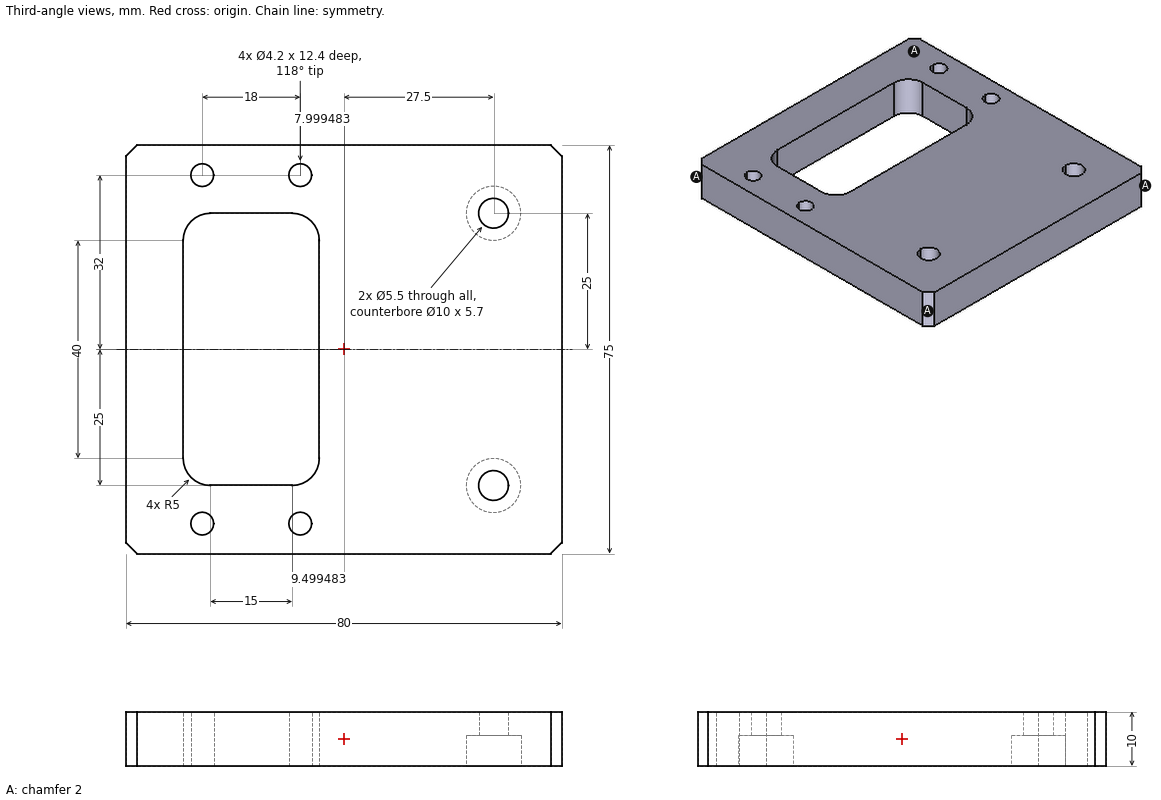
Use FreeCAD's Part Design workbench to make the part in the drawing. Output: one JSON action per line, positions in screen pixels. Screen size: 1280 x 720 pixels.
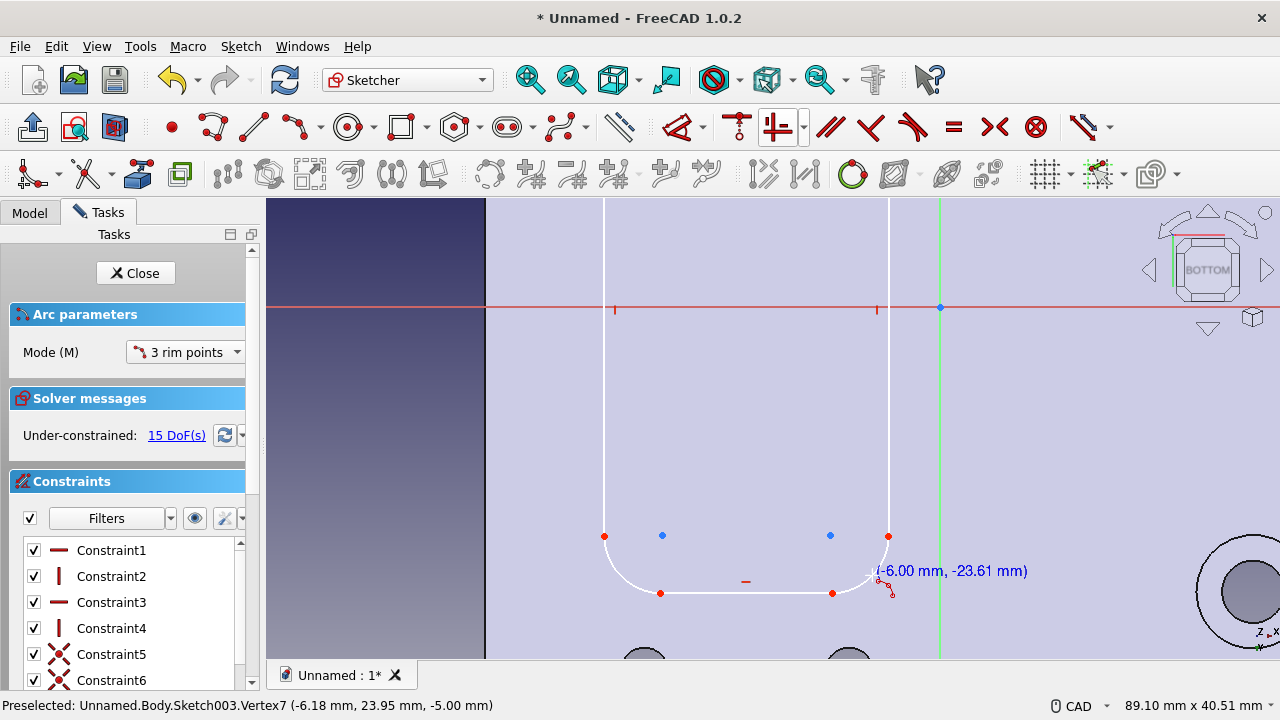
{"action": "scroll", "coordinate": [622, 576], "scroll_direction": "down", "scroll_amount": 3}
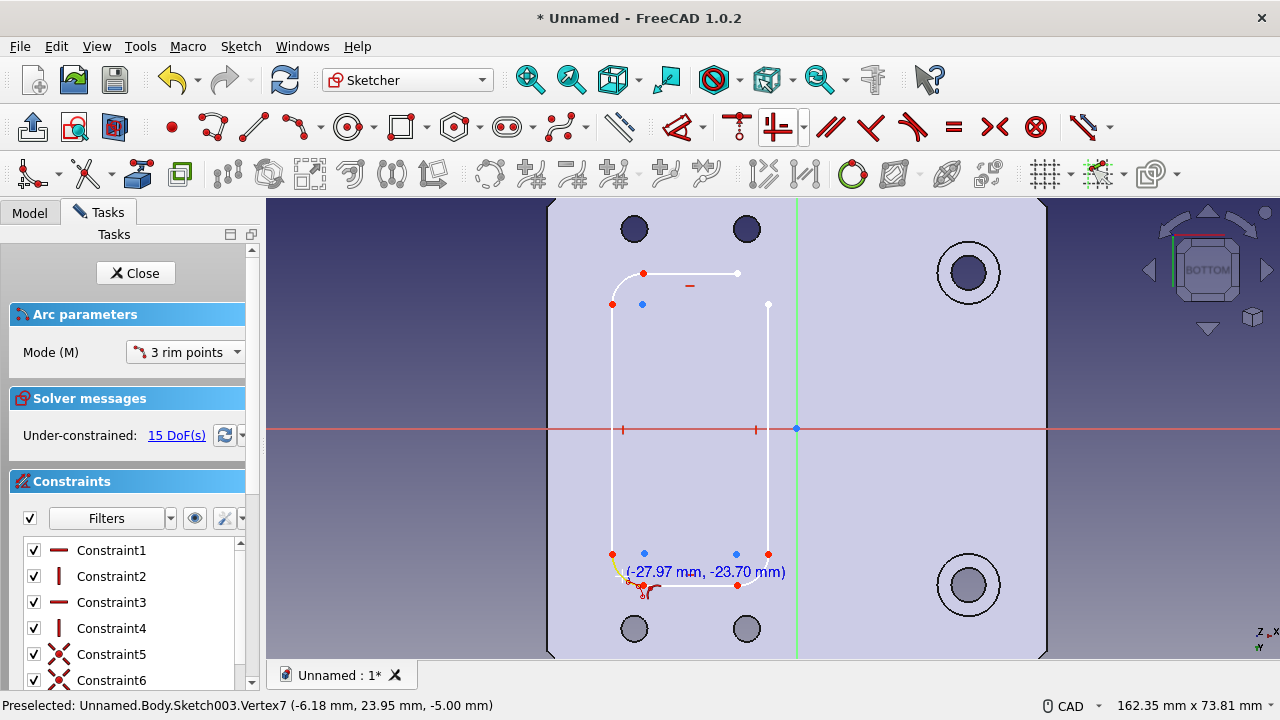
{"action": "left_click", "coordinate": [768, 305]}
{"action": "left_click", "coordinate": [737, 274]}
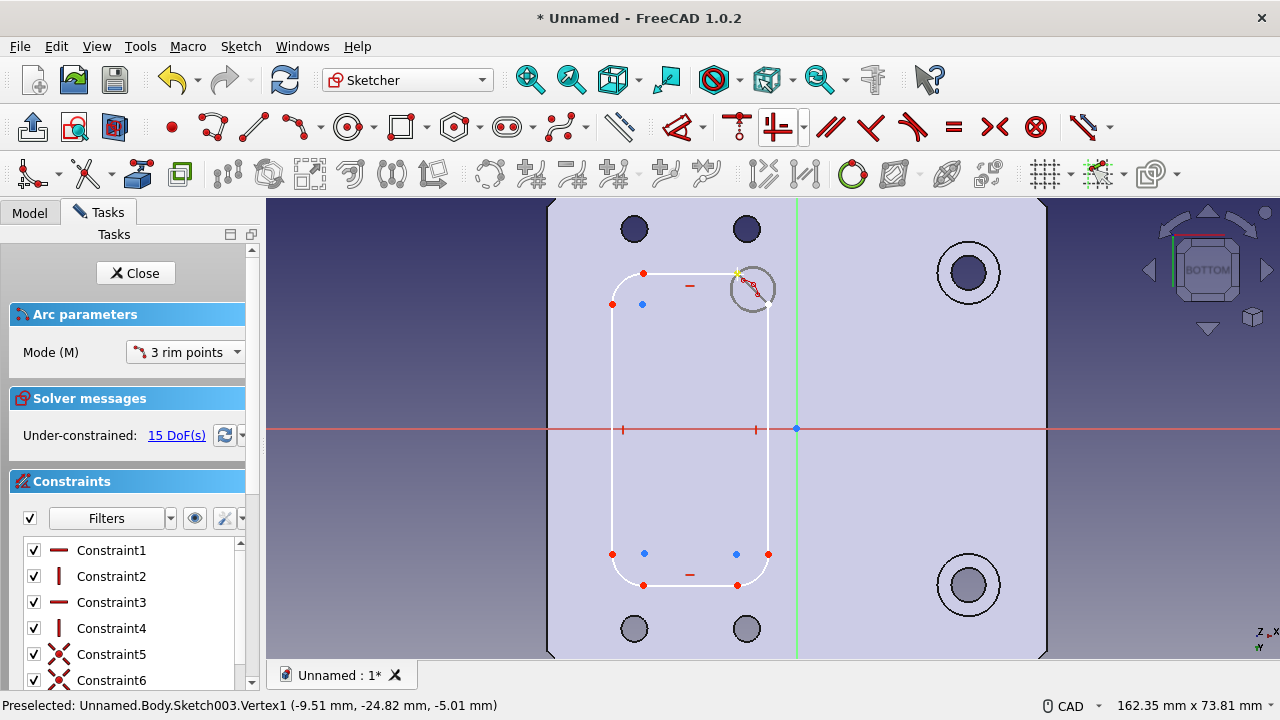
{"action": "scroll", "coordinate": [760, 282], "scroll_direction": "up", "scroll_amount": 3}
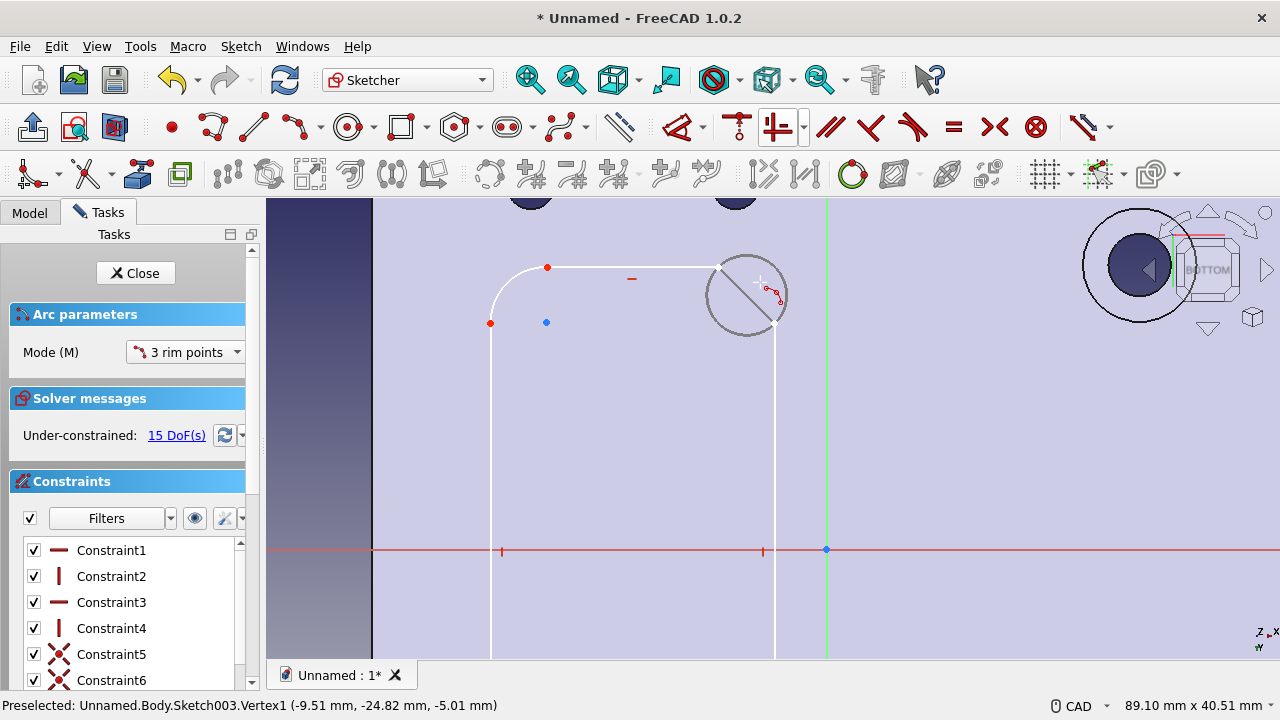
{"action": "left_click", "coordinate": [759, 282]}
{"action": "key", "text": "Escape"}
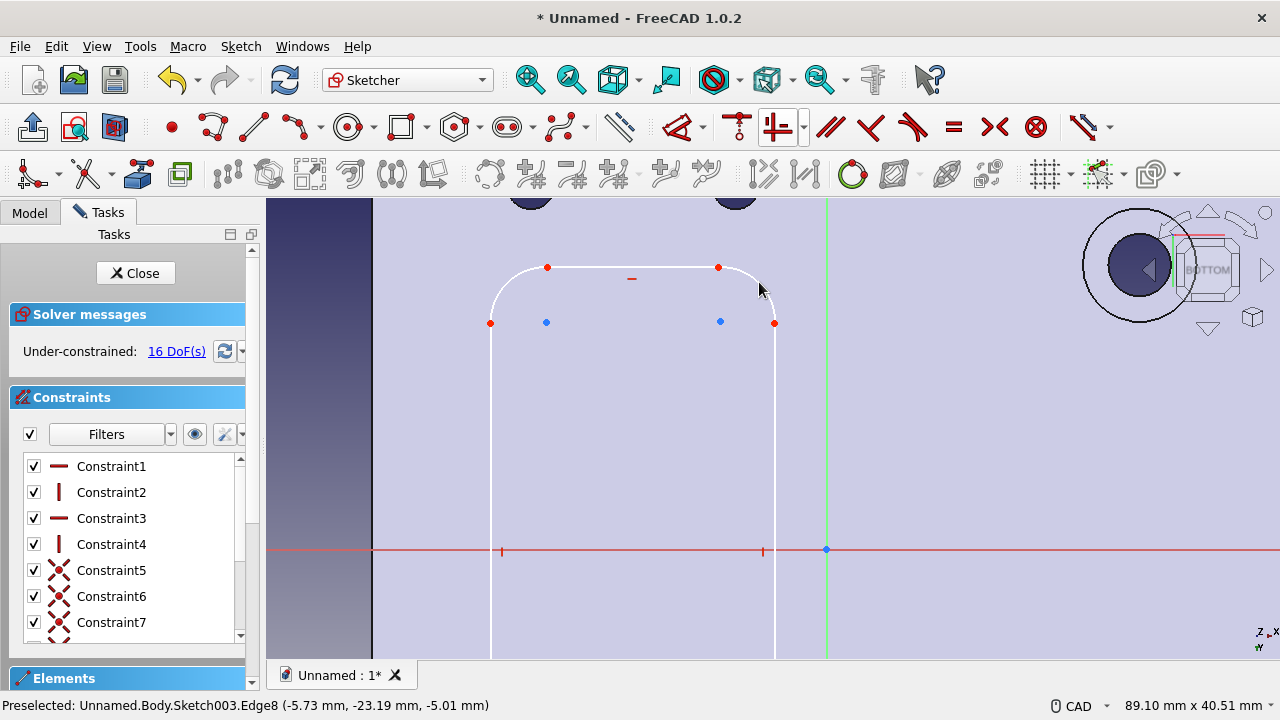
{"action": "left_click", "coordinate": [667, 267]}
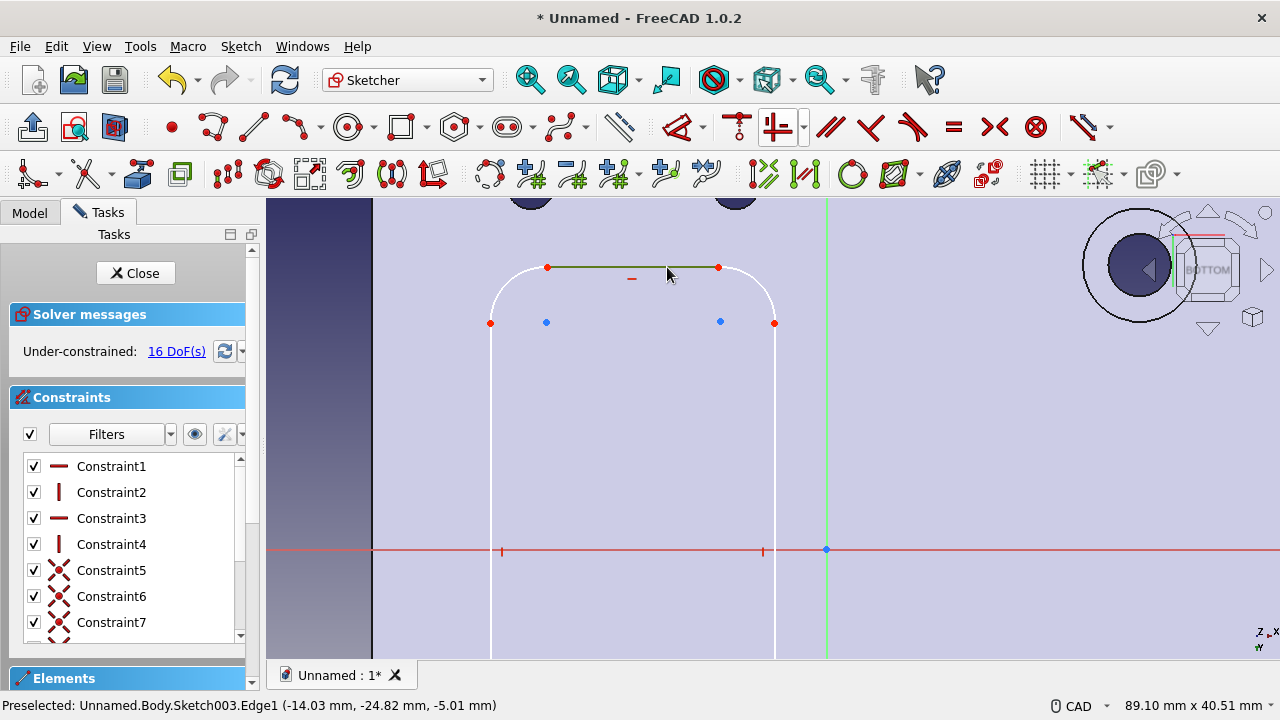
{"action": "left_click", "coordinate": [521, 273]}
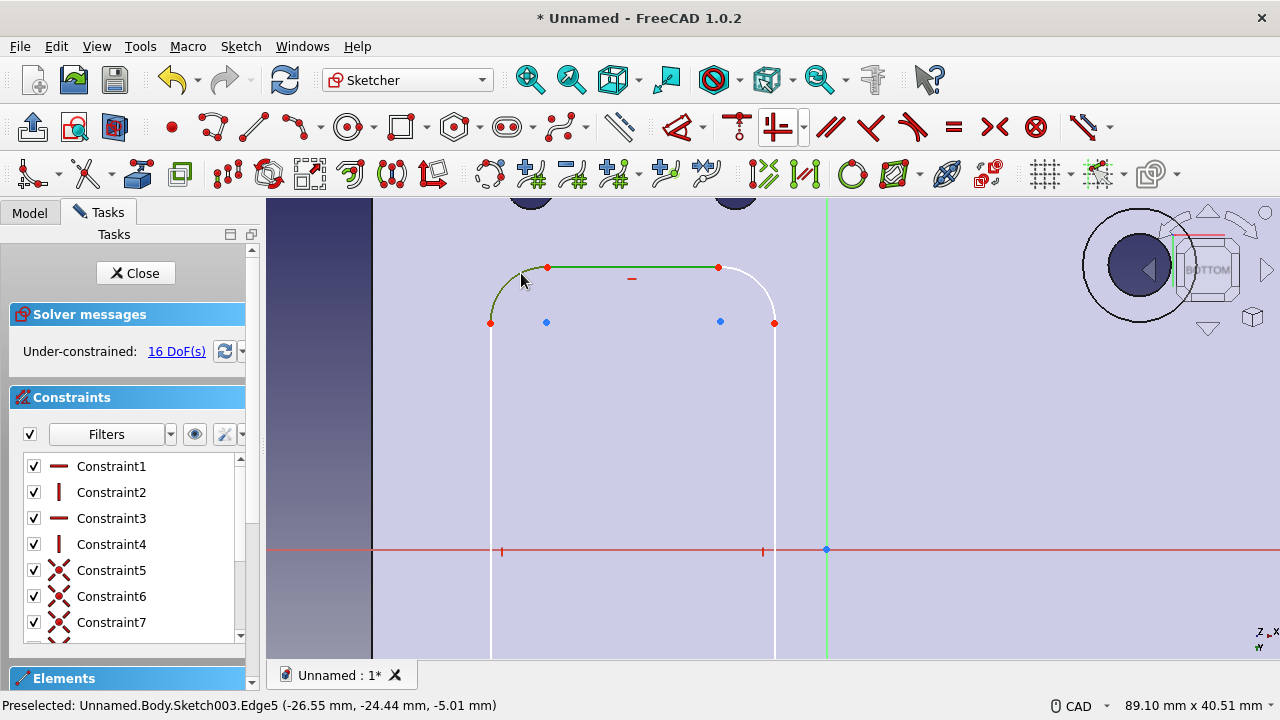
{"action": "key", "text": "t"}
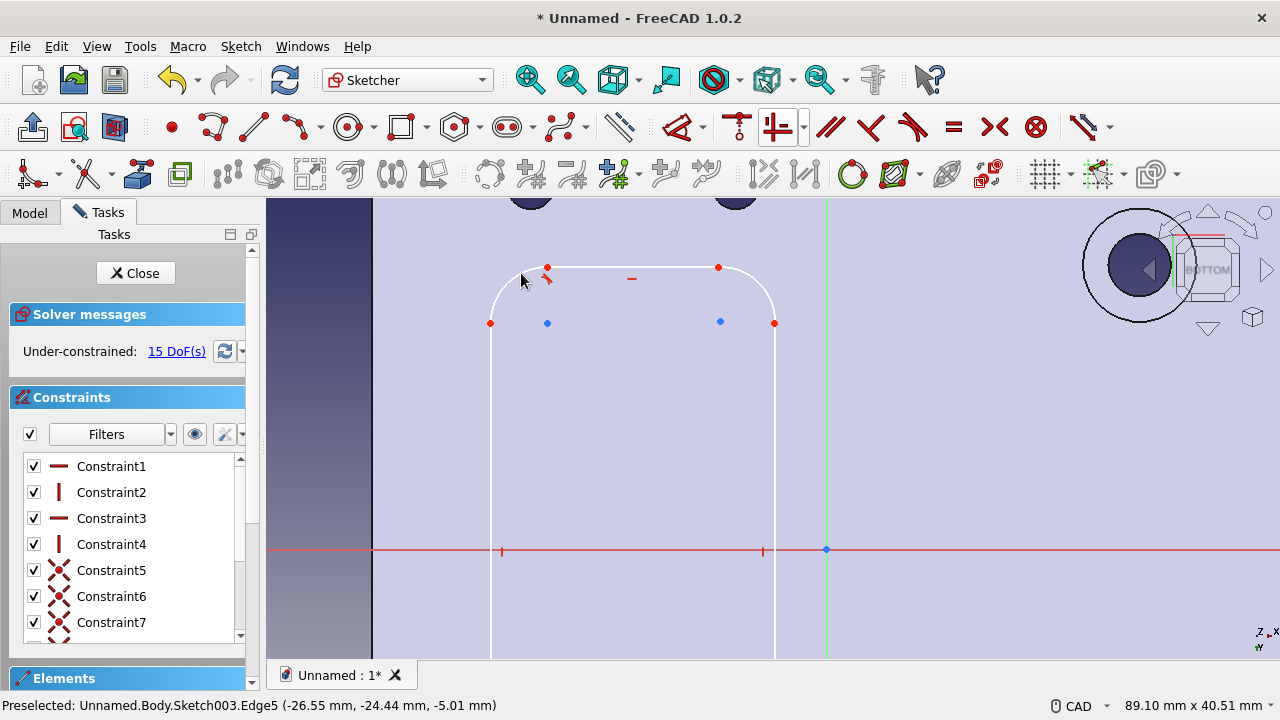
{"action": "left_click", "coordinate": [667, 267]}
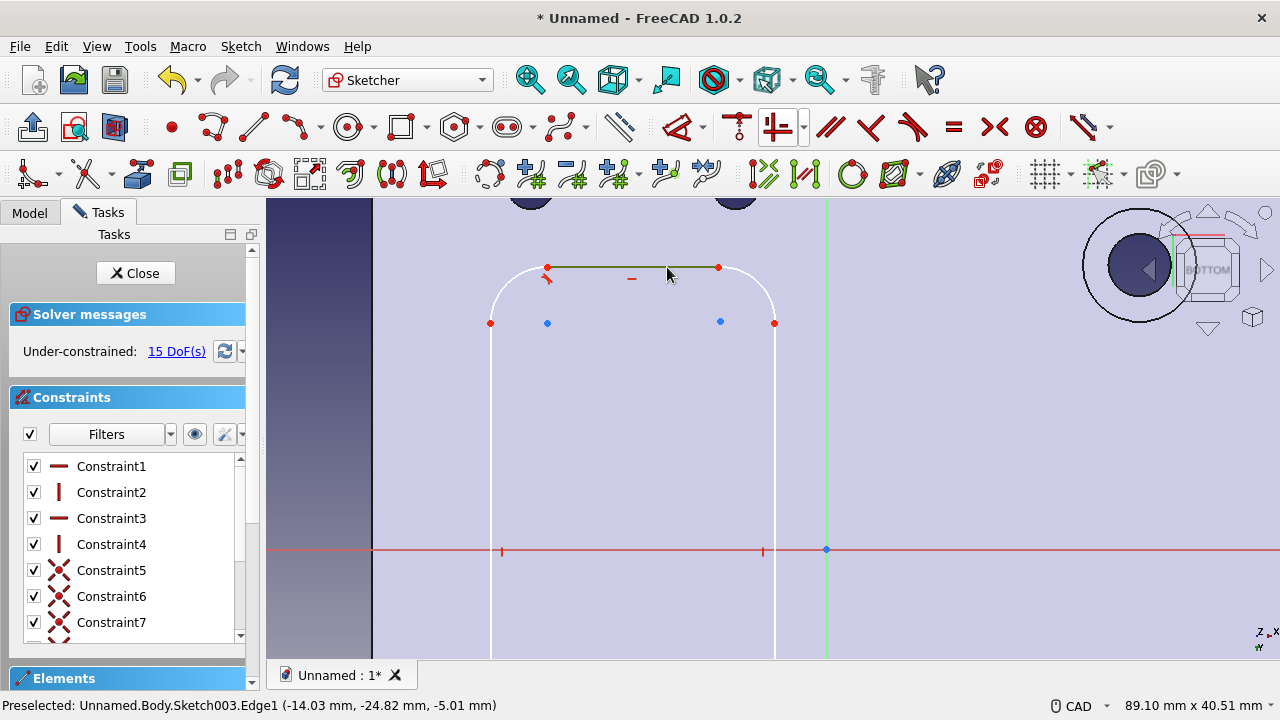
{"action": "left_click", "coordinate": [769, 298]}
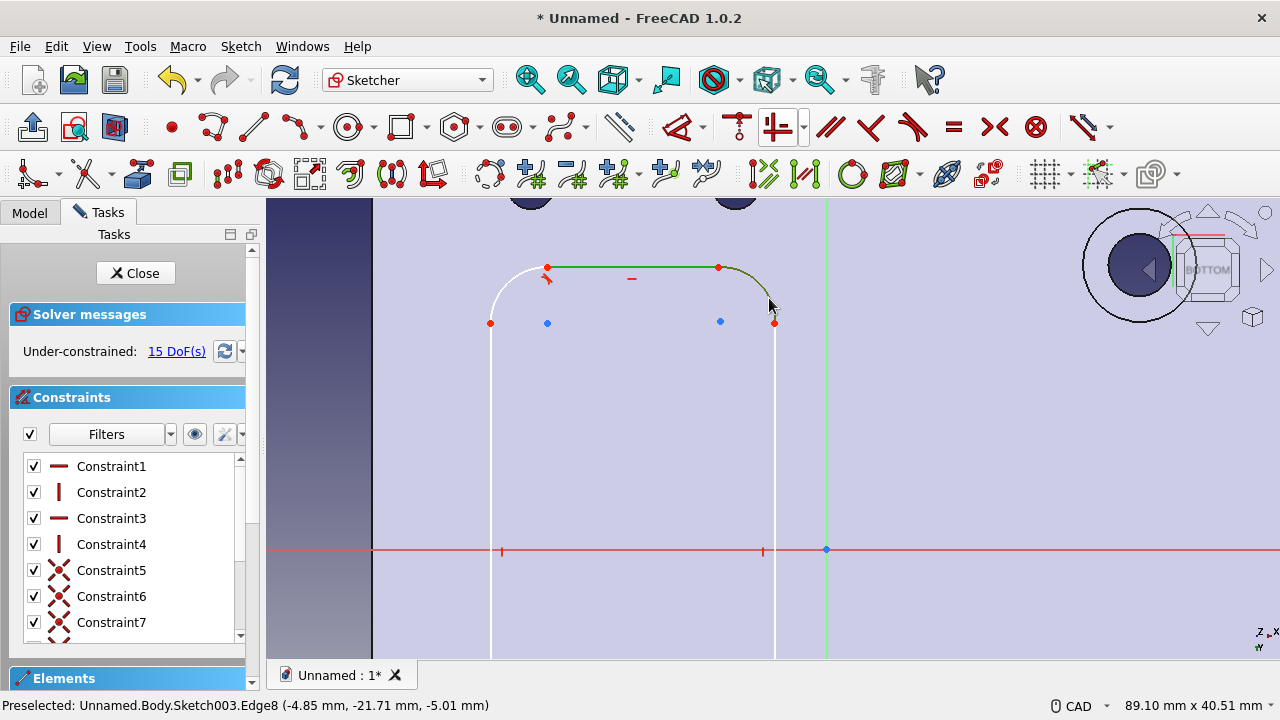
{"action": "key", "text": "t"}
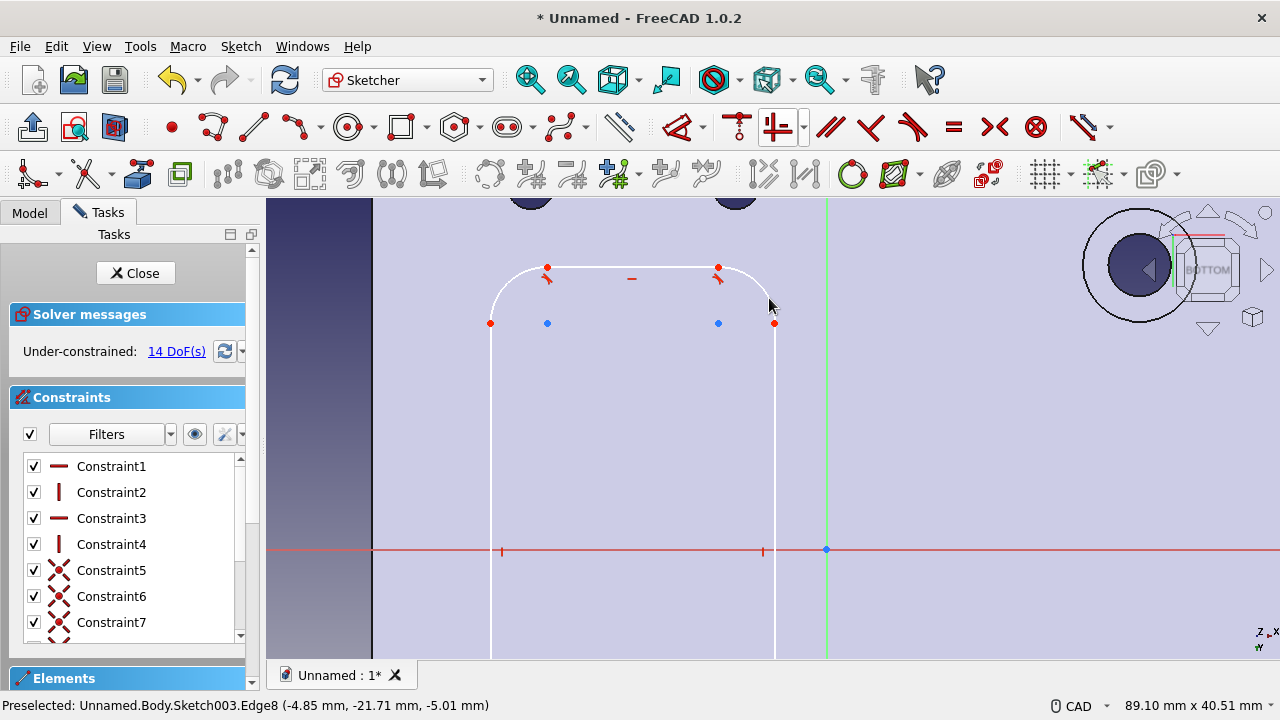
{"action": "left_click", "coordinate": [491, 460]}